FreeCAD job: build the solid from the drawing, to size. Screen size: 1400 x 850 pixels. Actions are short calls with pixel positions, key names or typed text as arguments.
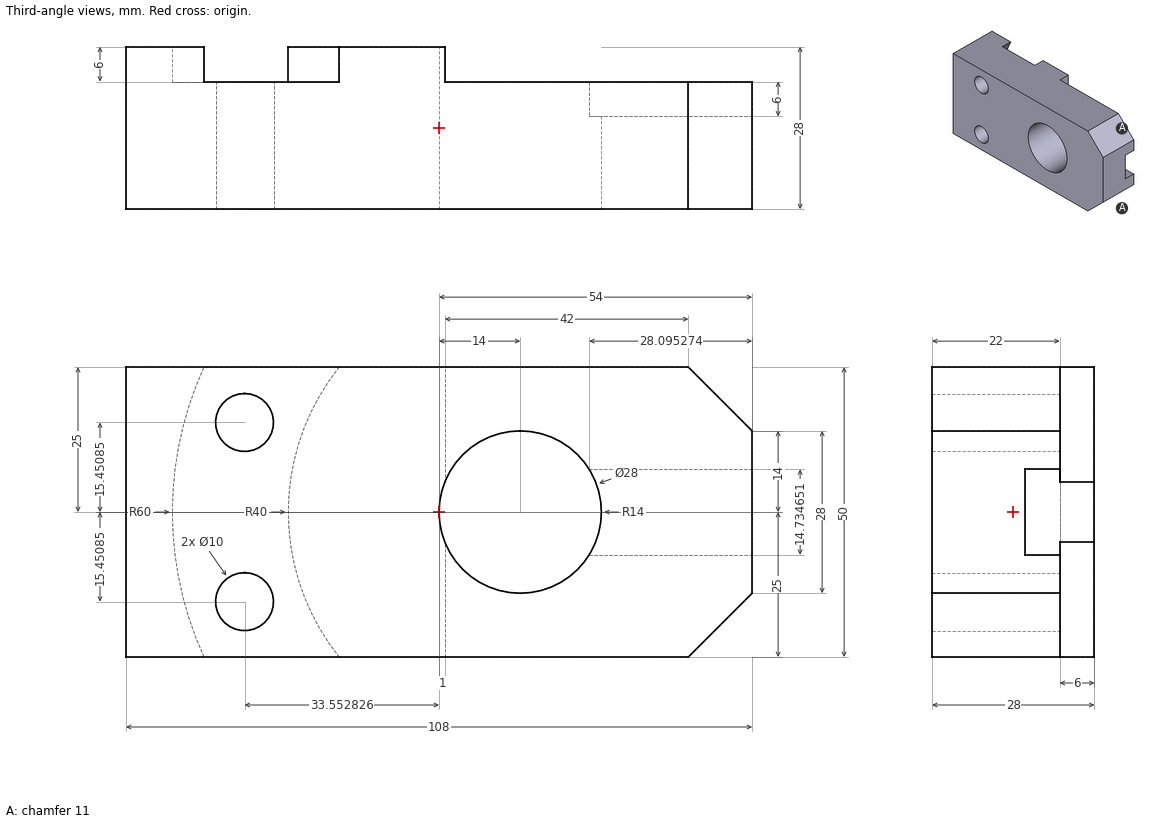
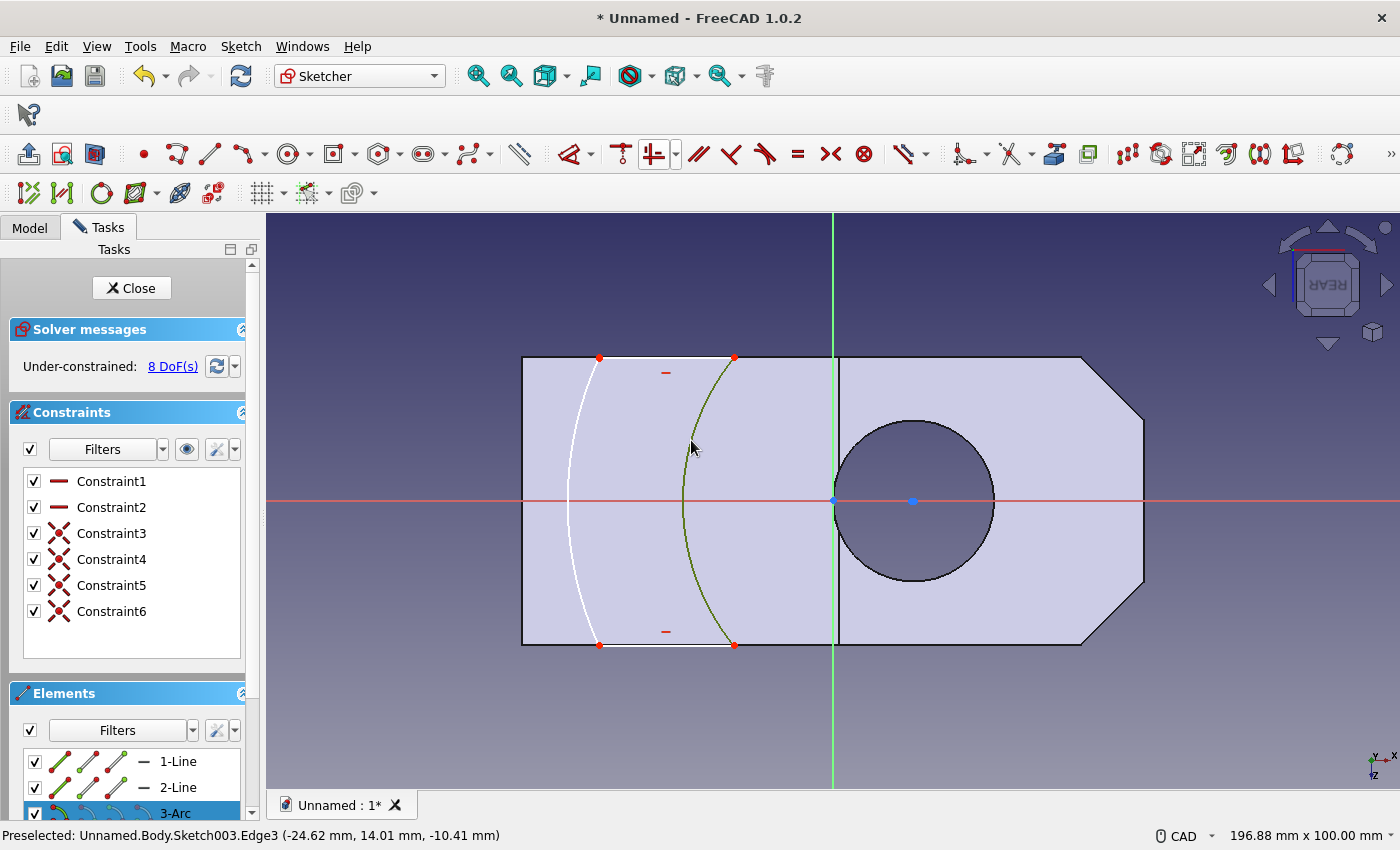
click(573, 443)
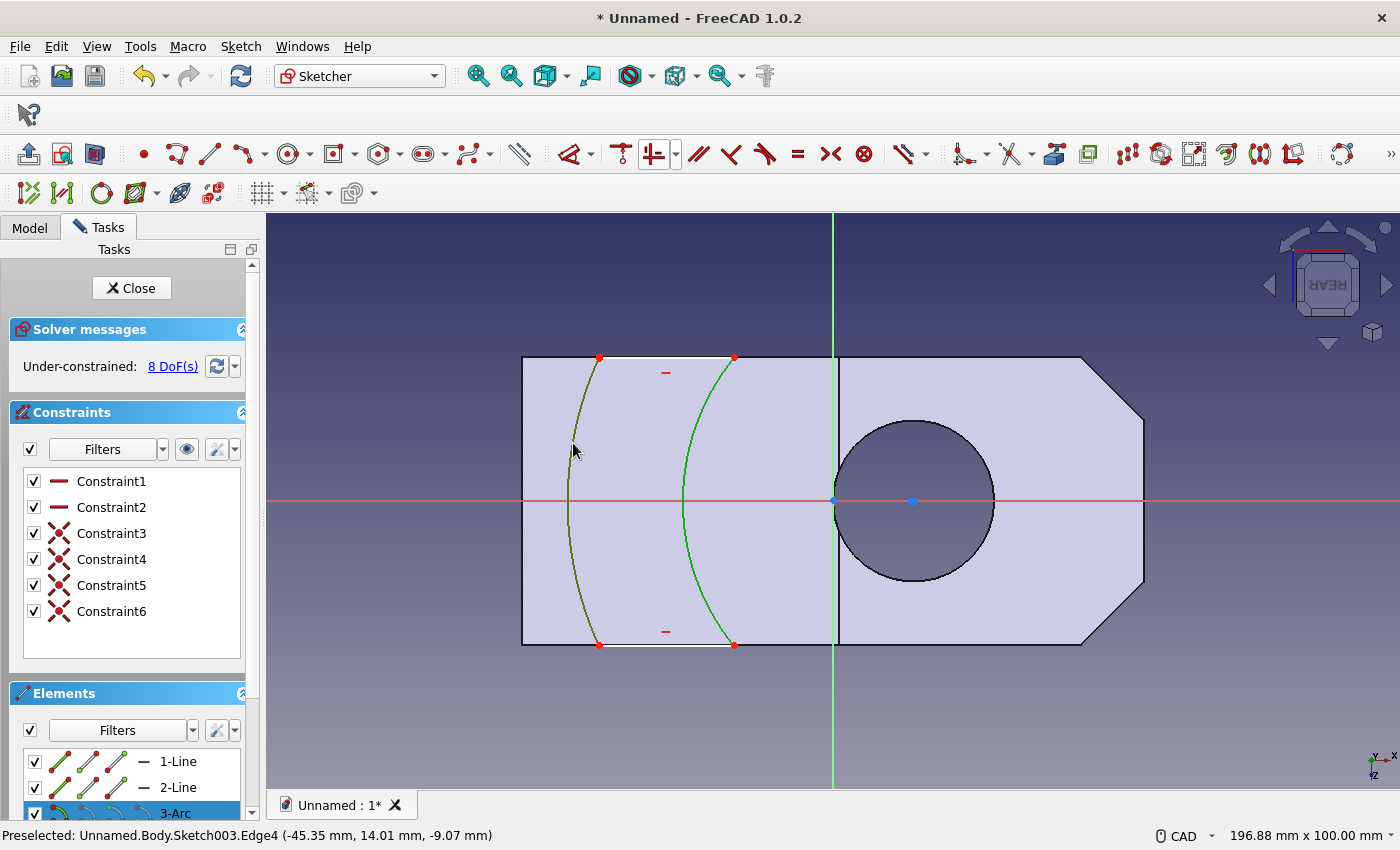
click(621, 154)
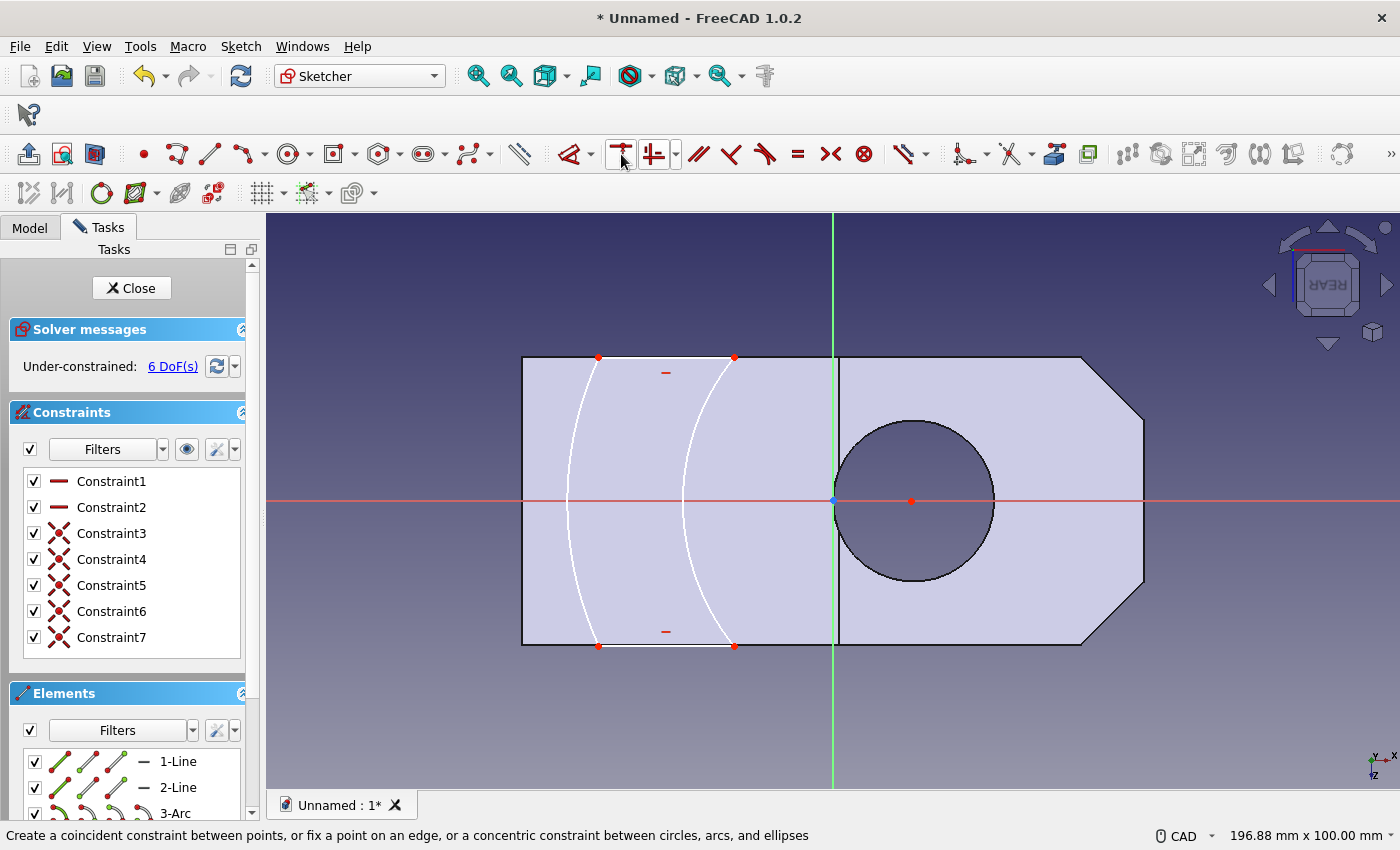
click(911, 502)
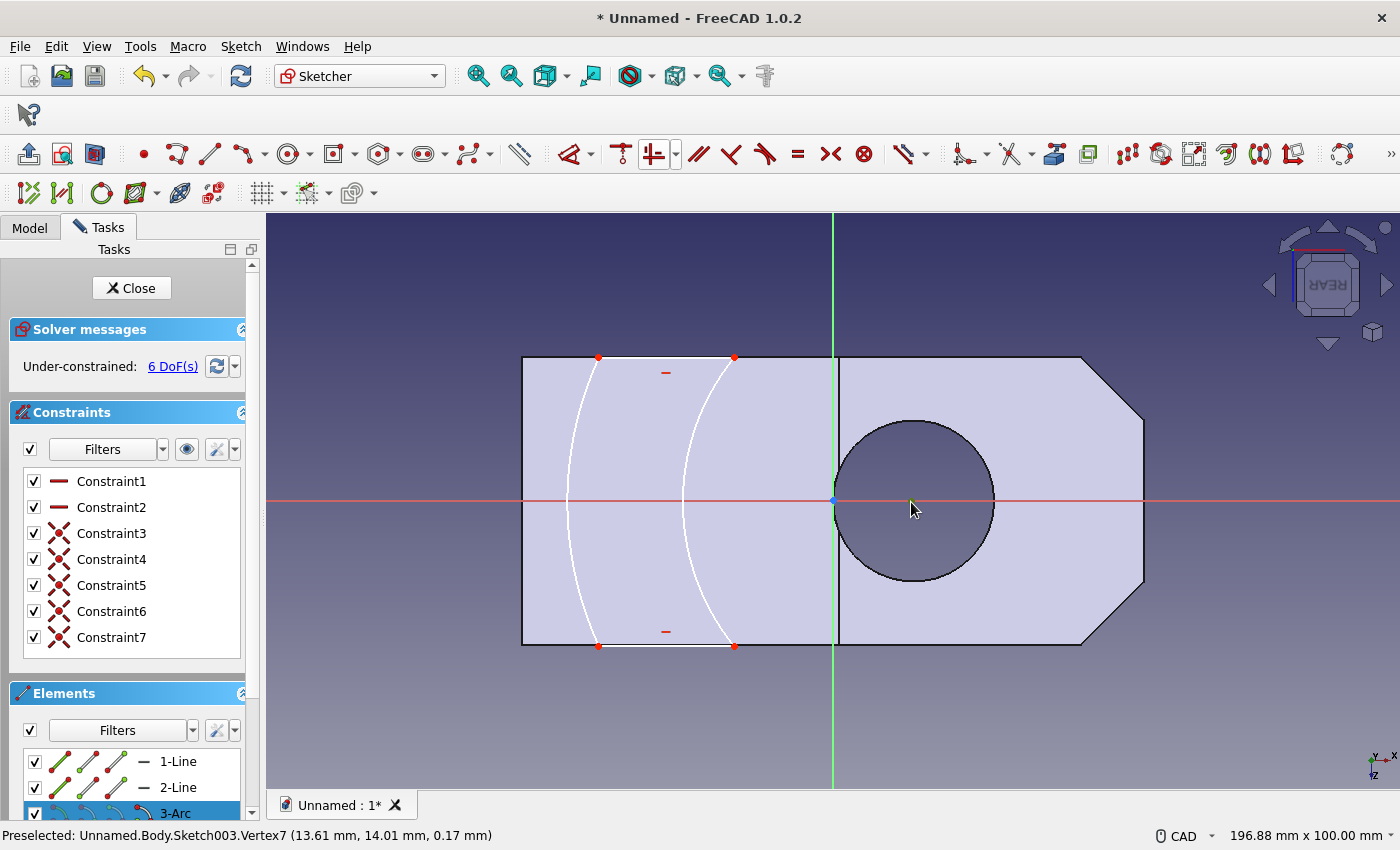
click(361, 501)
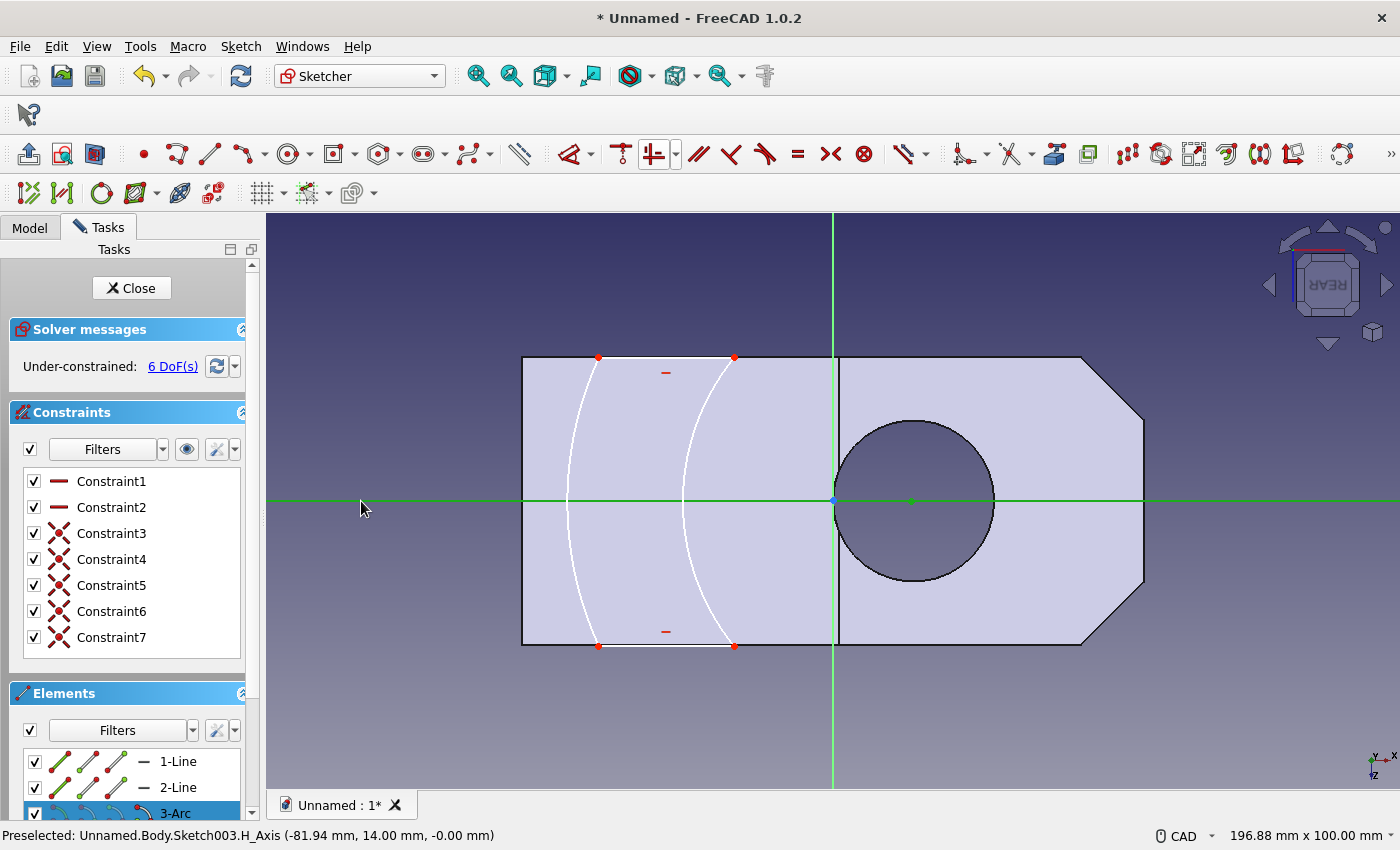
key(c)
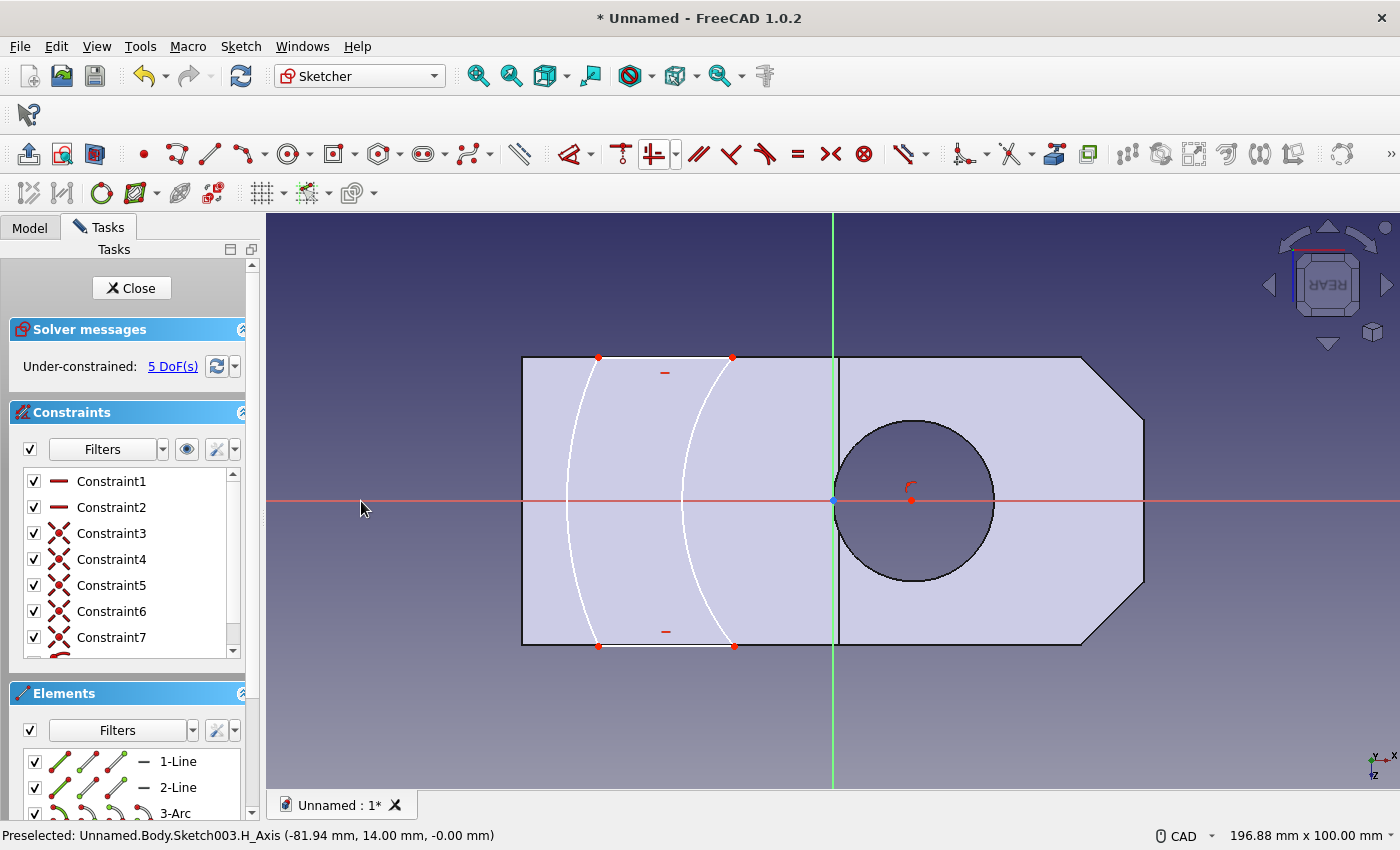
click(568, 154)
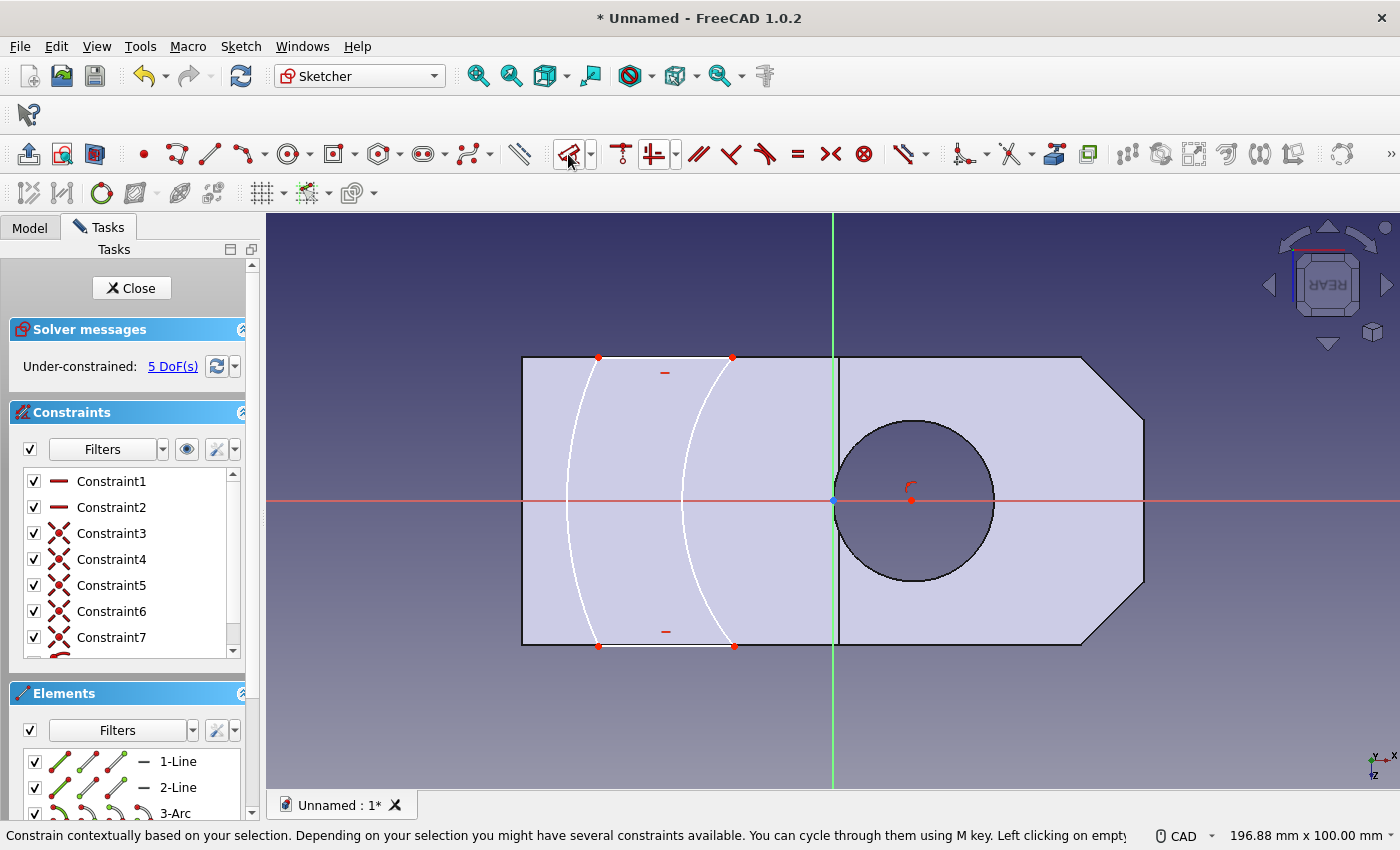
click(690, 441)
click(659, 433)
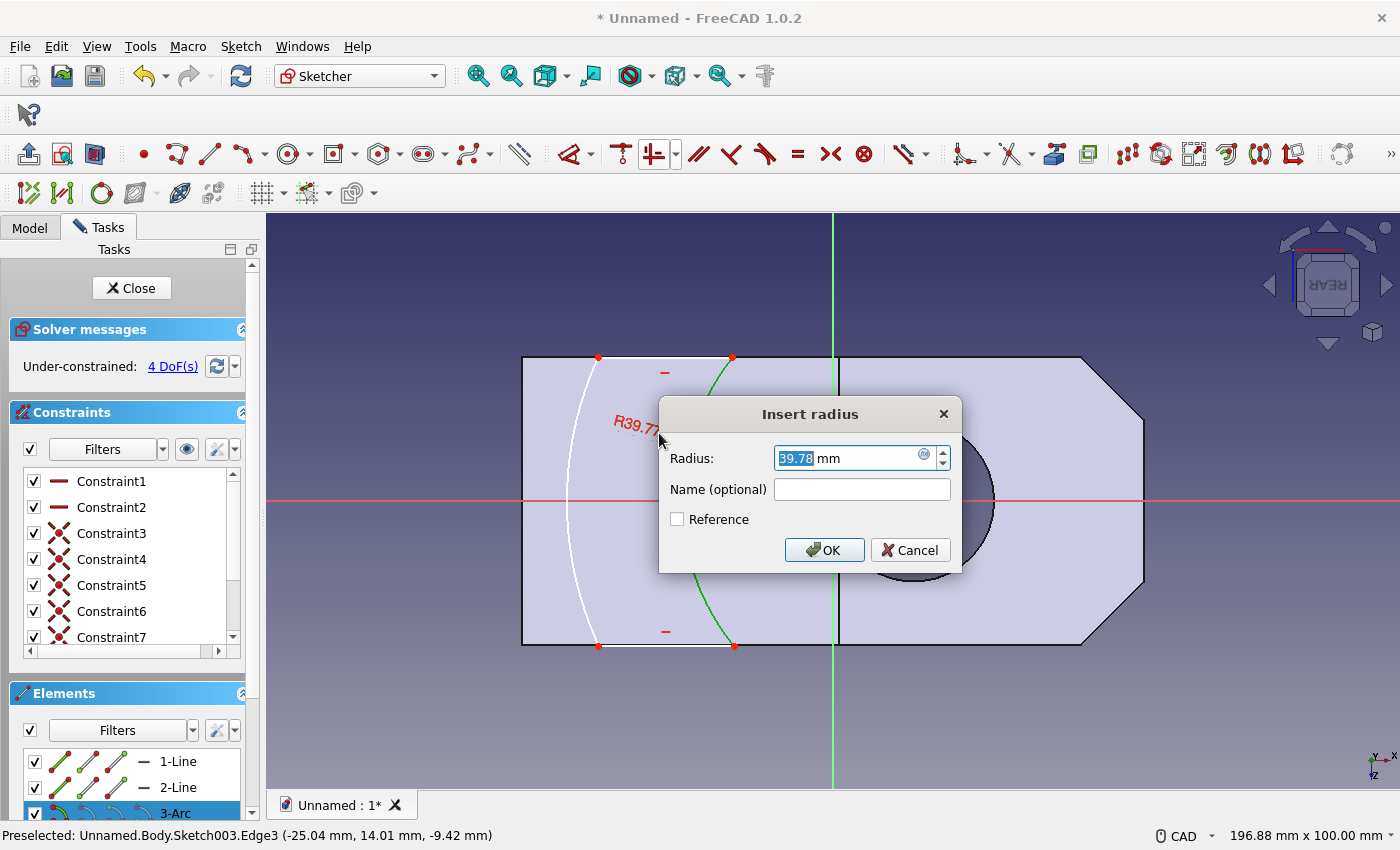
text(40)
key(Return)